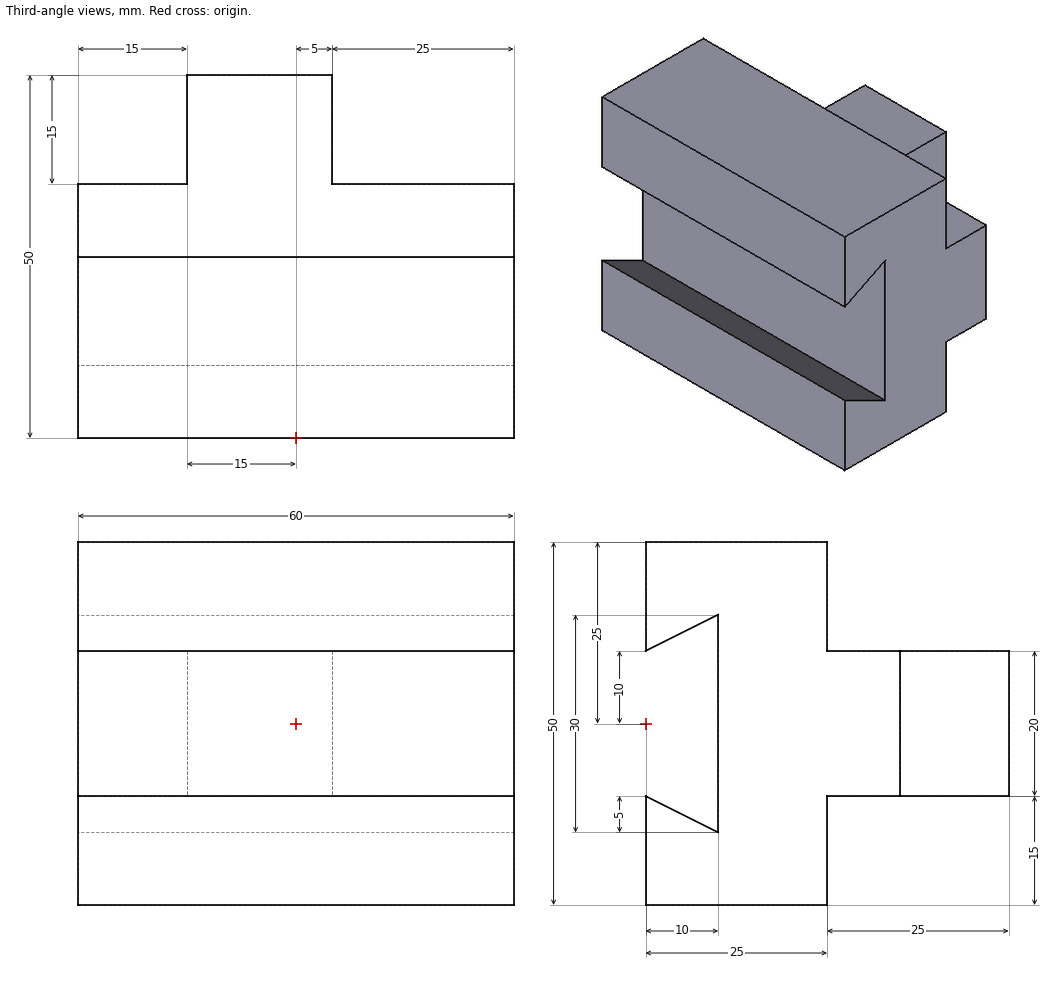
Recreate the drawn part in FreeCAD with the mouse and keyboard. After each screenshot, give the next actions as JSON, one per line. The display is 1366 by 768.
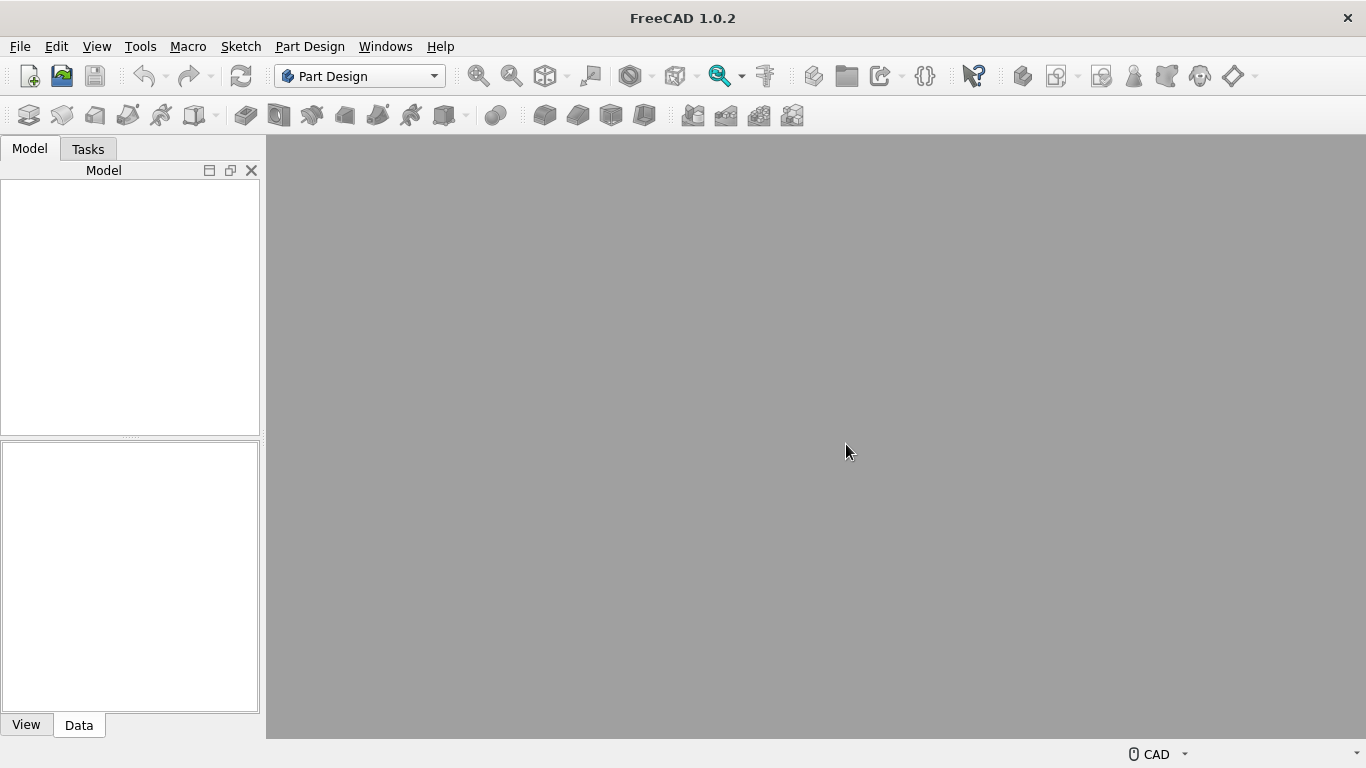
{"action": "key", "text": "ctrl+n"}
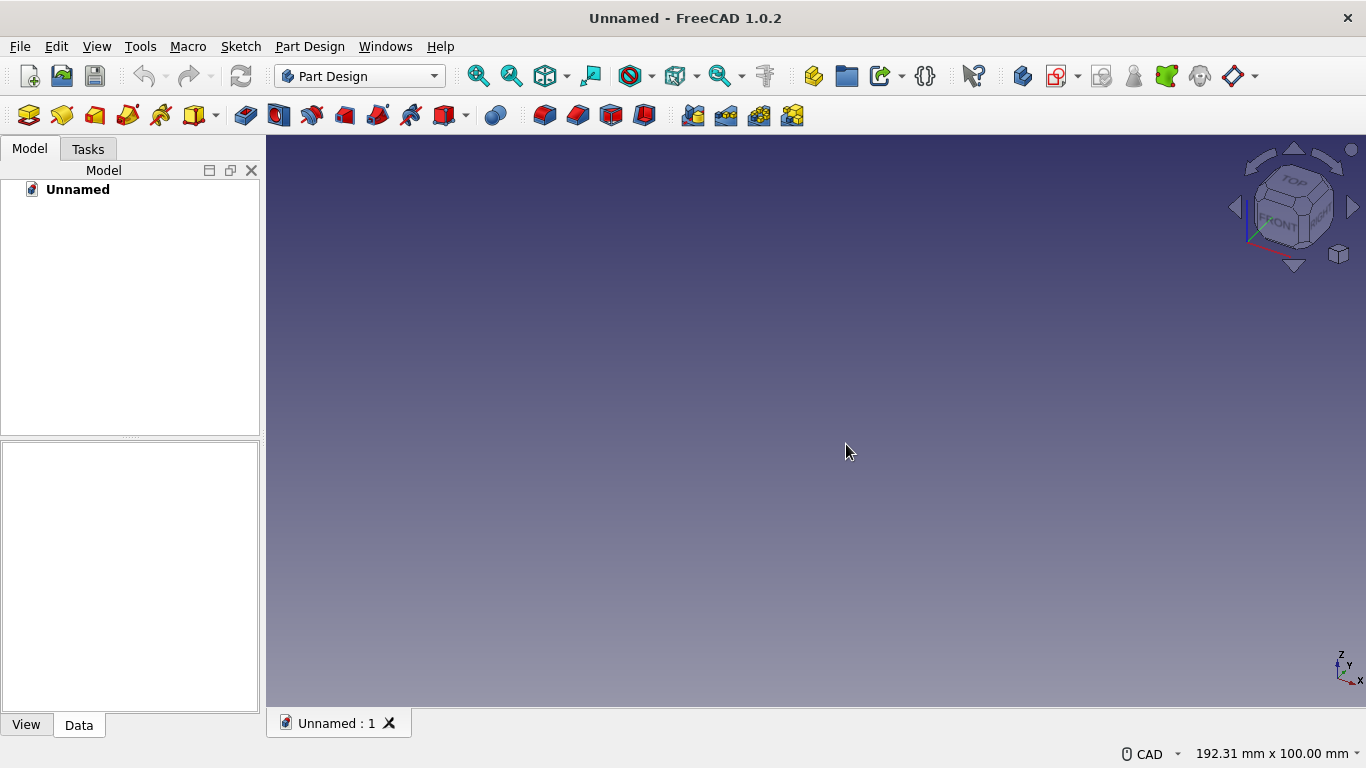
{"action": "left_click", "coordinate": [1056, 76]}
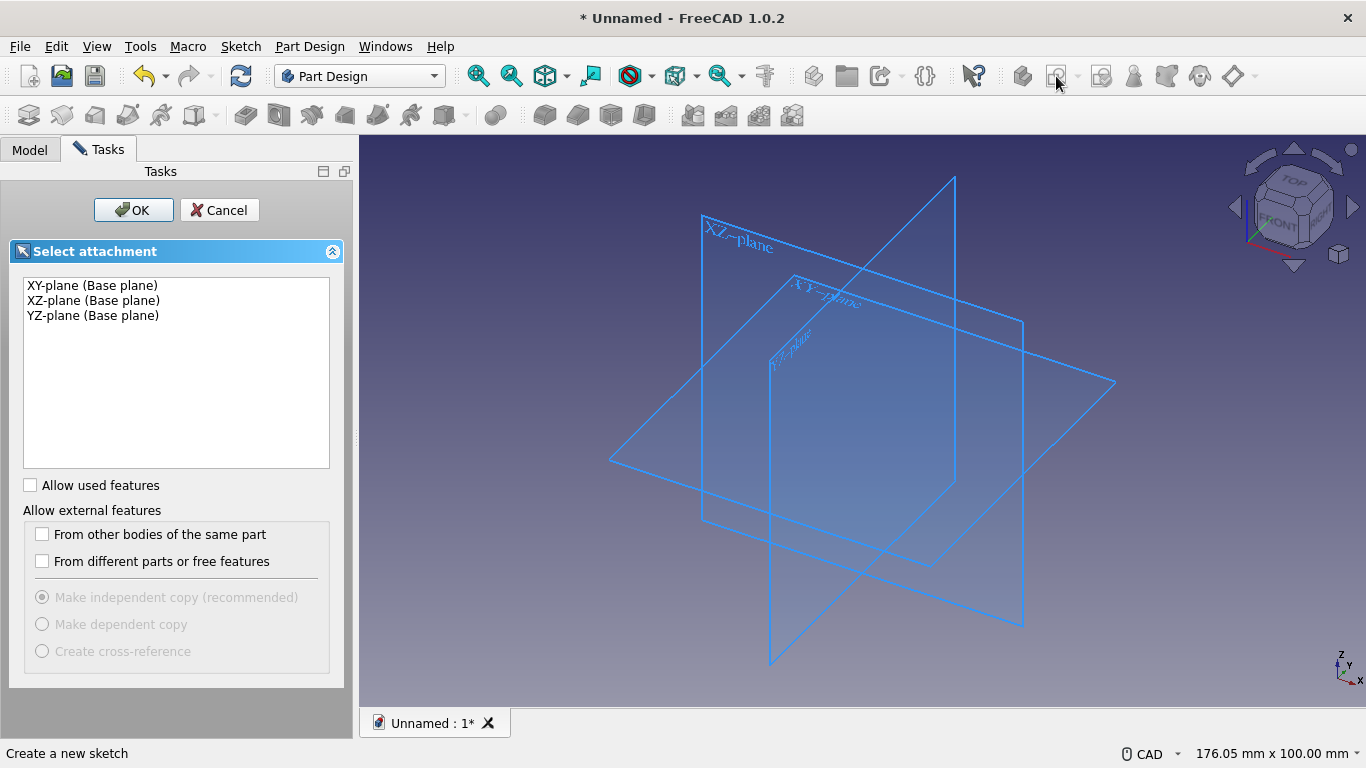
{"action": "left_click", "coordinate": [84, 316]}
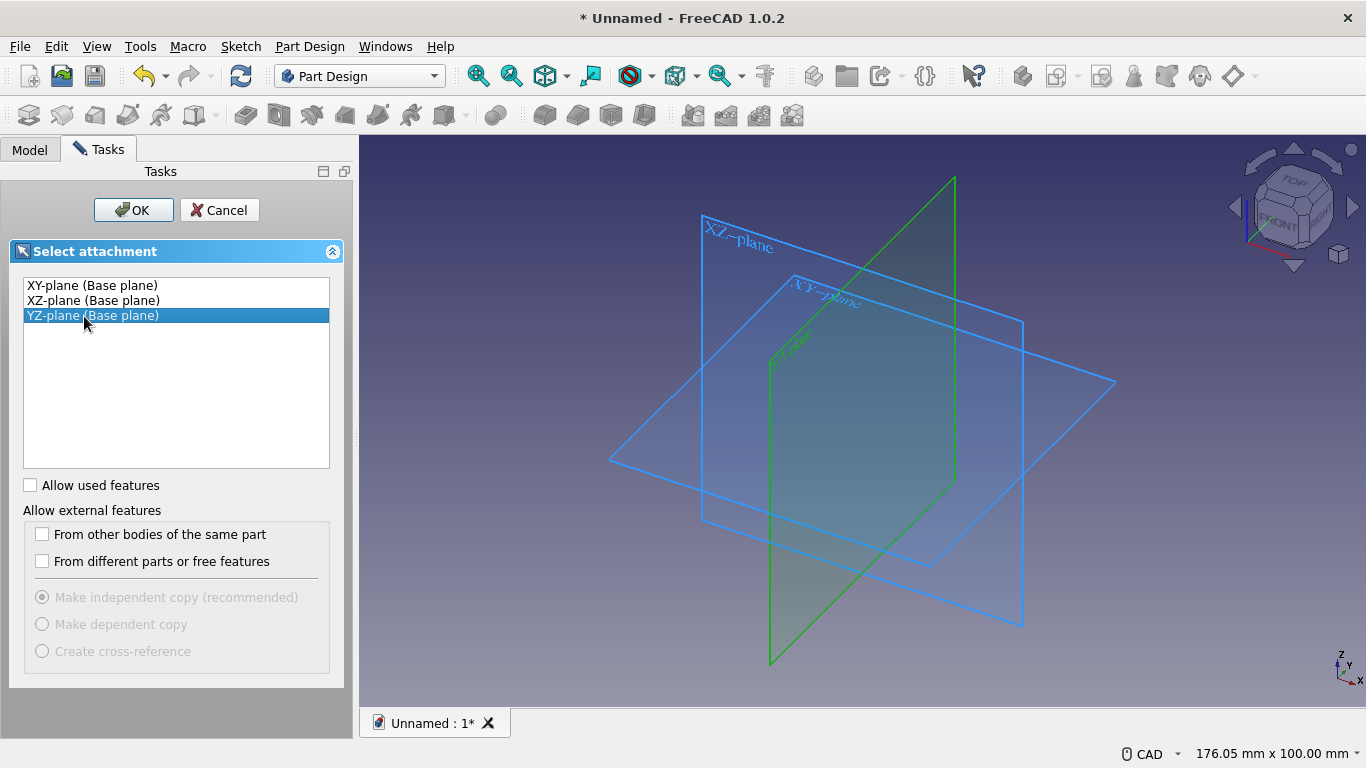
{"action": "left_click", "coordinate": [134, 210]}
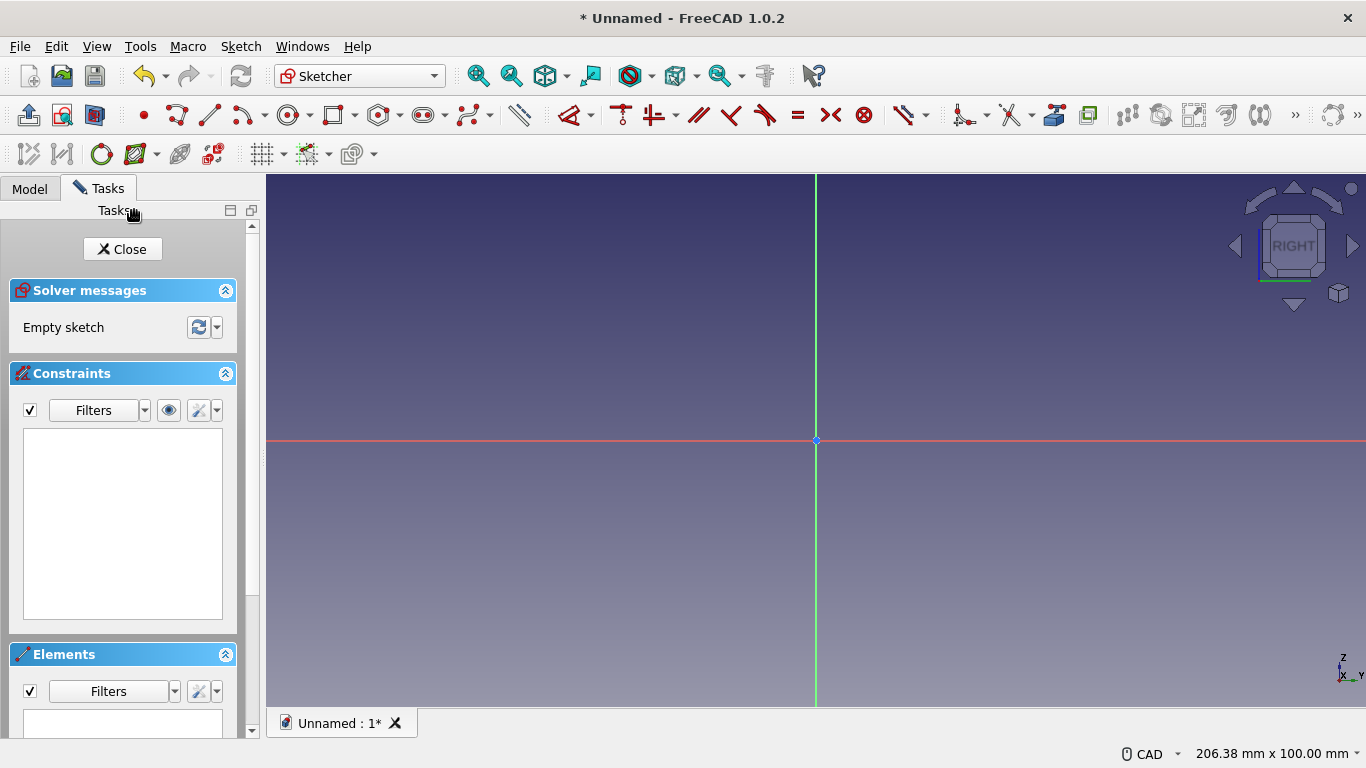
{"action": "left_click", "coordinate": [177, 116]}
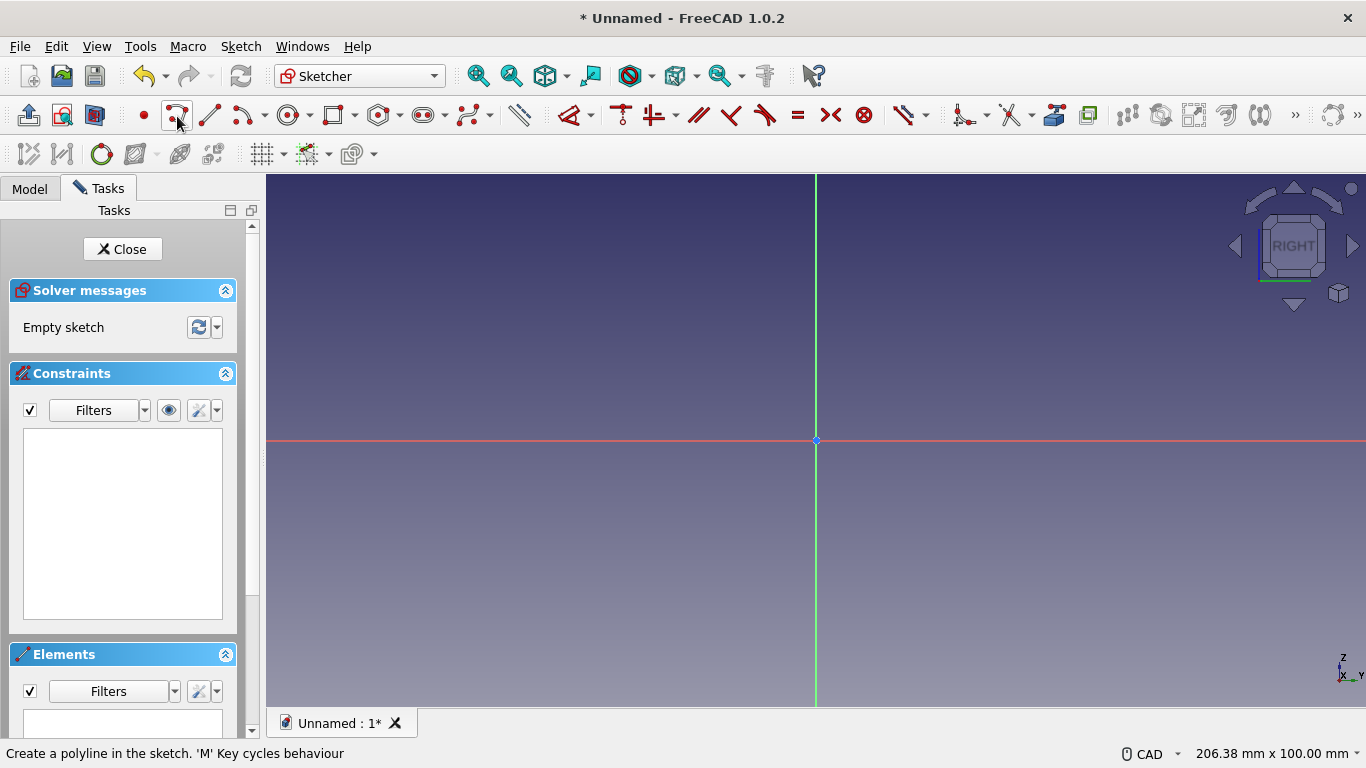
{"action": "left_click", "coordinate": [816, 307]}
{"action": "left_click", "coordinate": [825, 574]}
{"action": "left_click", "coordinate": [949, 574]}
{"action": "left_click", "coordinate": [949, 494]}
{"action": "left_click", "coordinate": [1082, 494]}
{"action": "left_click", "coordinate": [1082, 387]}
{"action": "left_click", "coordinate": [949, 387]}
{"action": "left_click", "coordinate": [949, 307]}
{"action": "left_click", "coordinate": [816, 308]}
{"action": "key", "text": "Escape"}
{"action": "key", "text": "Escape"}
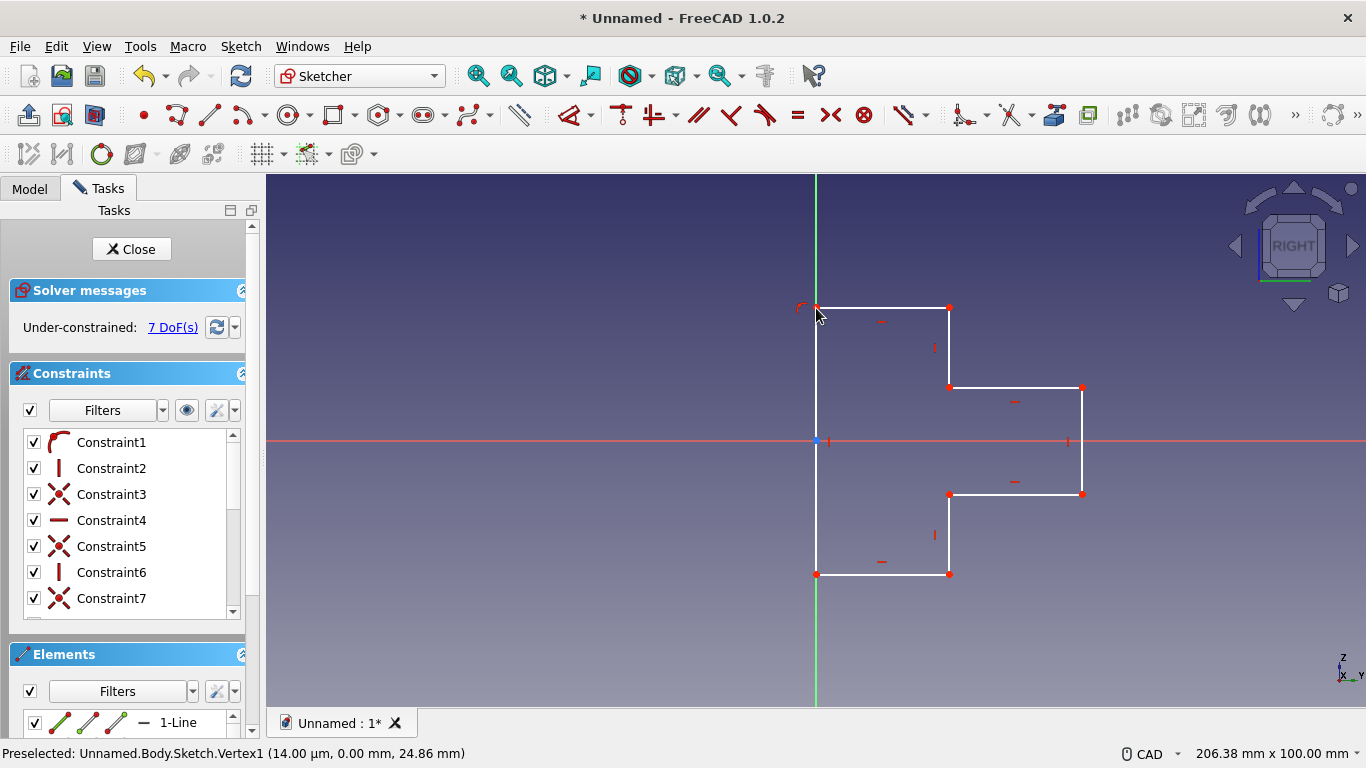
{"action": "left_click", "coordinate": [816, 388]}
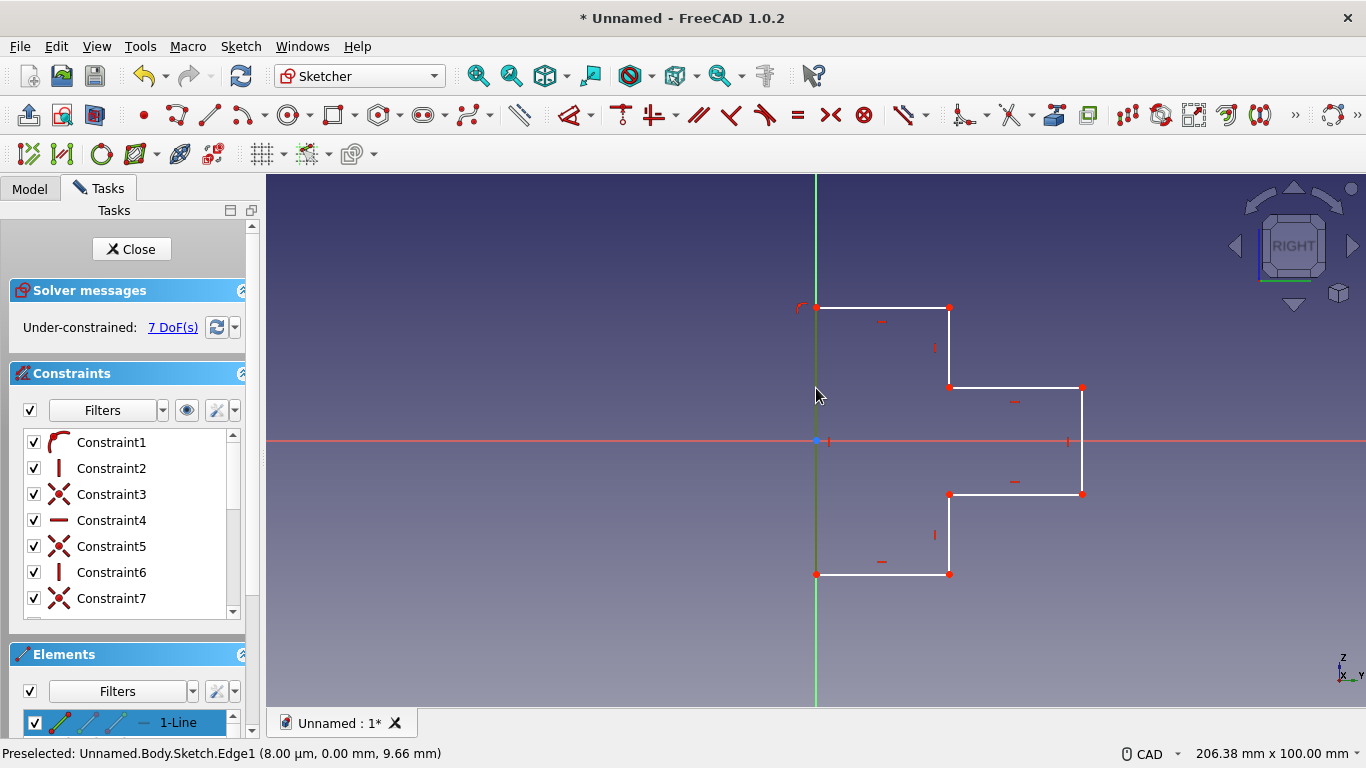
{"action": "key", "text": "i"}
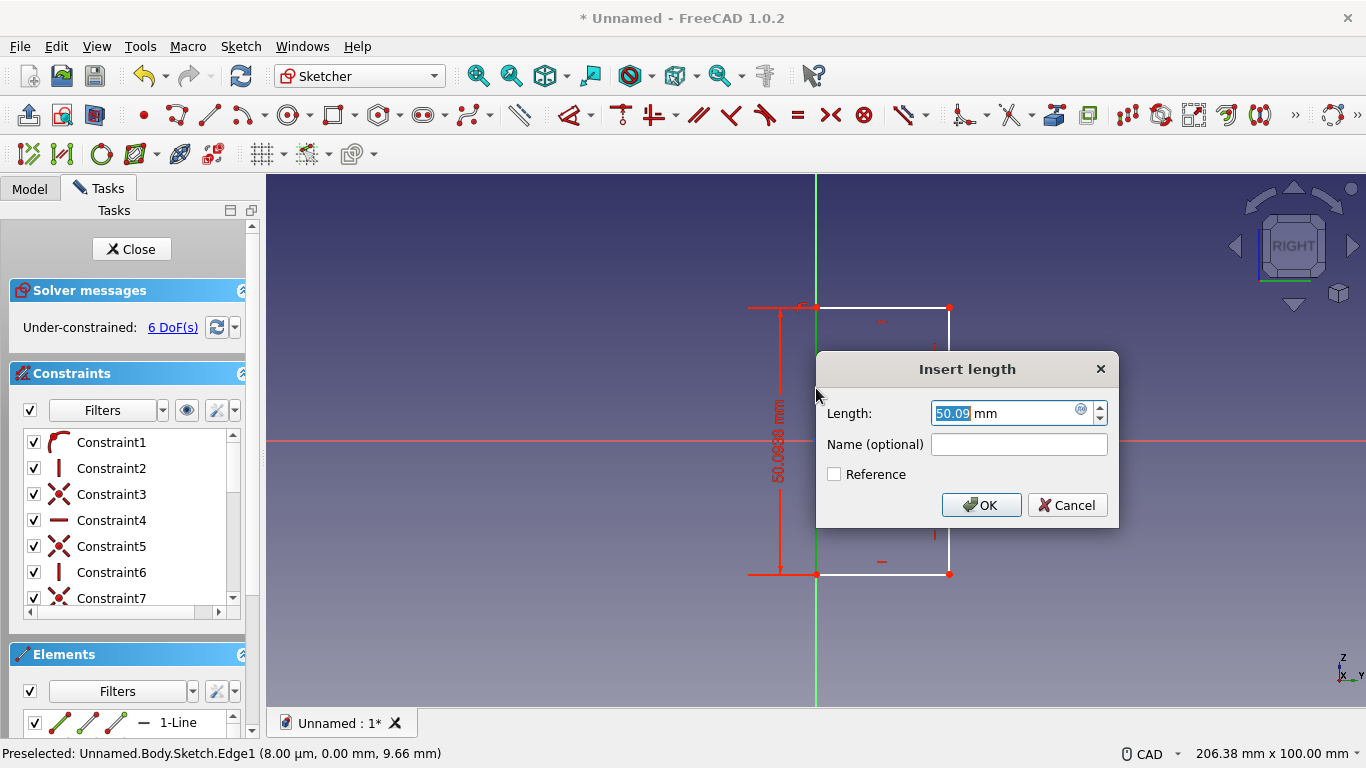
{"action": "type", "text": "50"}
{"action": "key", "text": "Return"}